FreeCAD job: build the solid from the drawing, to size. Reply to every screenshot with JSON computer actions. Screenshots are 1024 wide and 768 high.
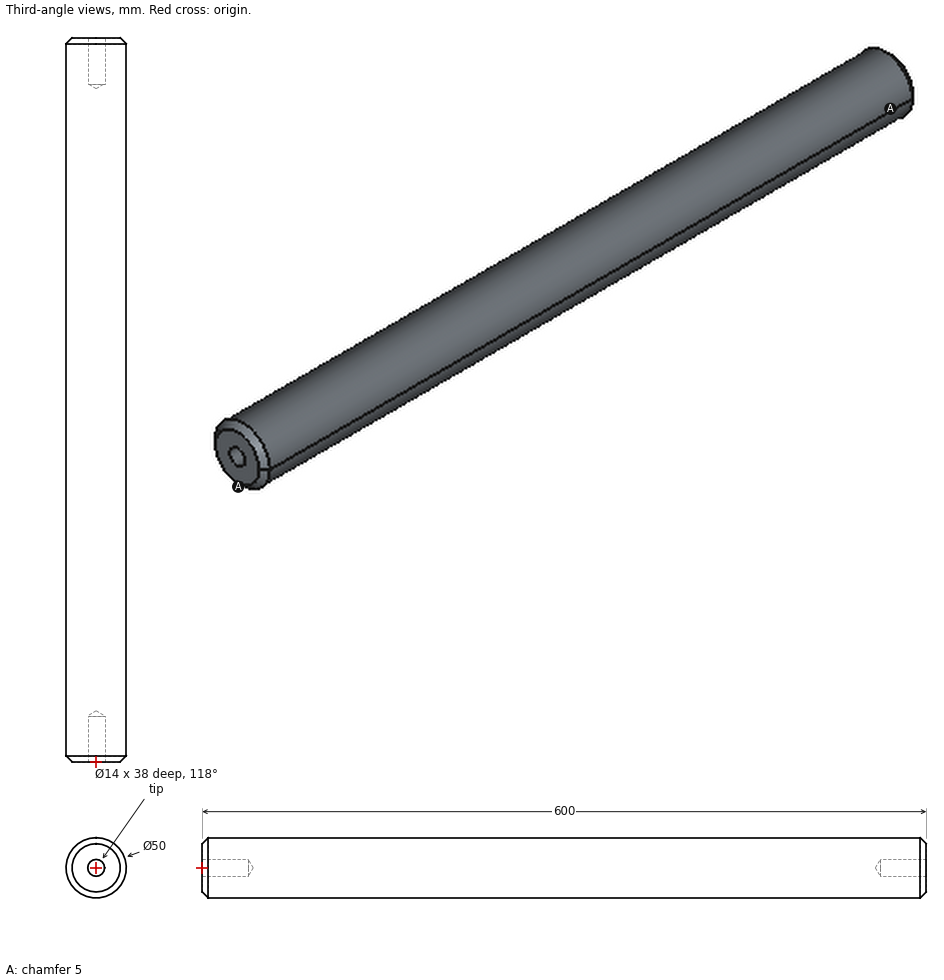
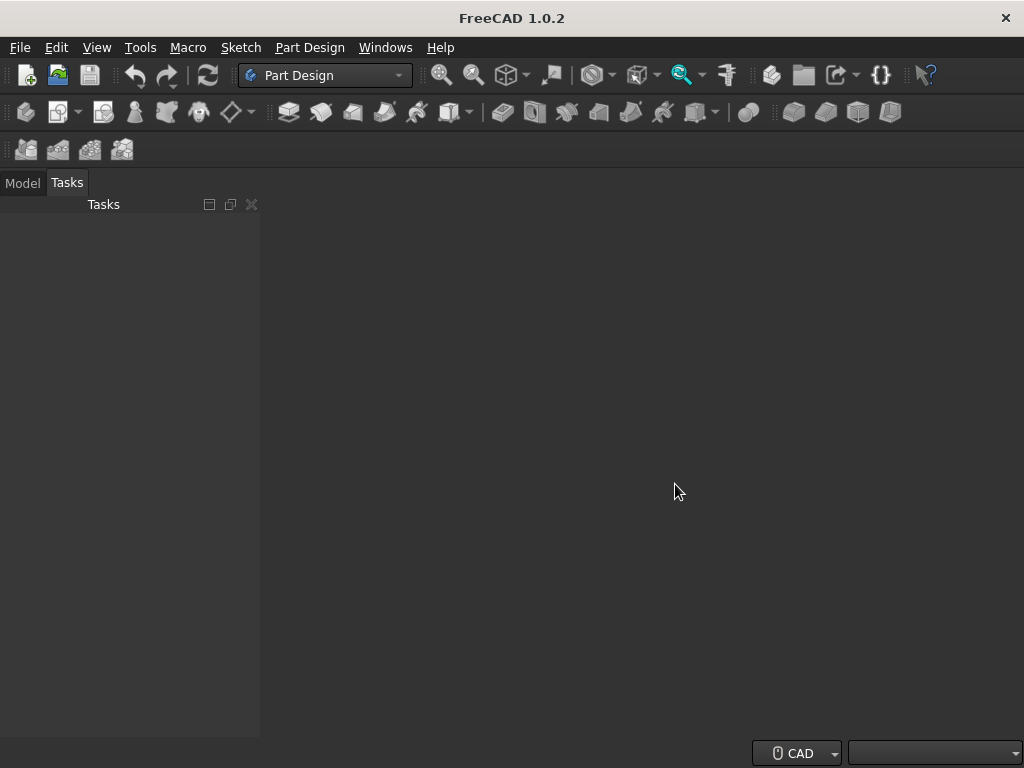
{"action": "left_click", "coordinate": [26, 76]}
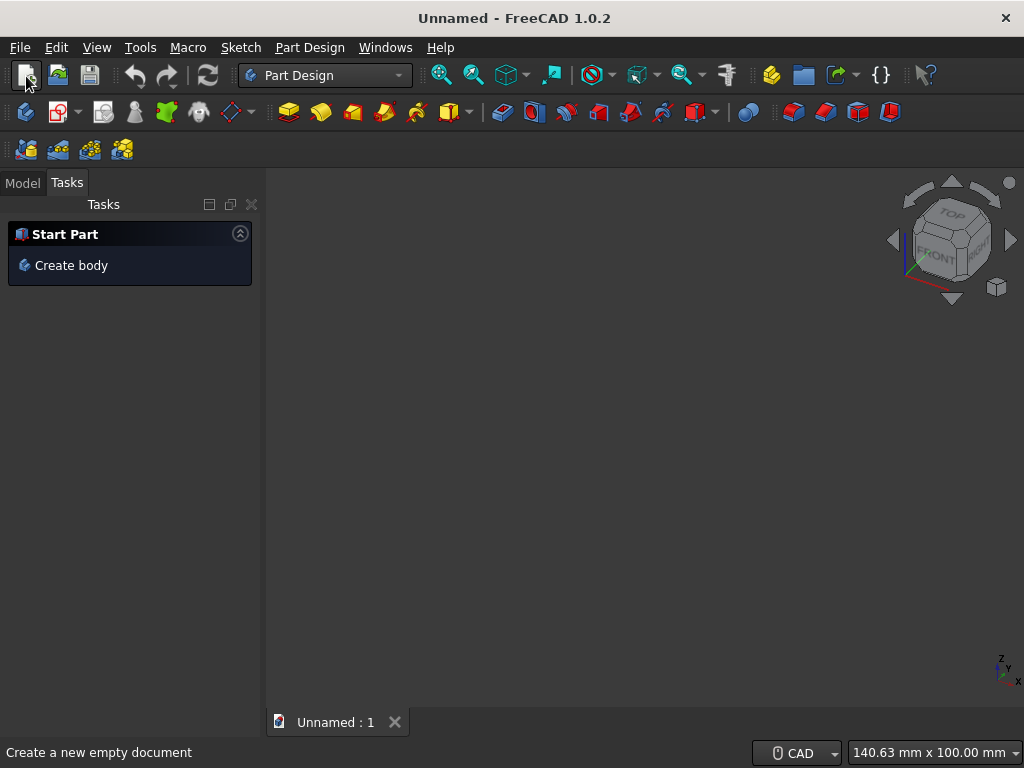
{"action": "left_click", "coordinate": [58, 112]}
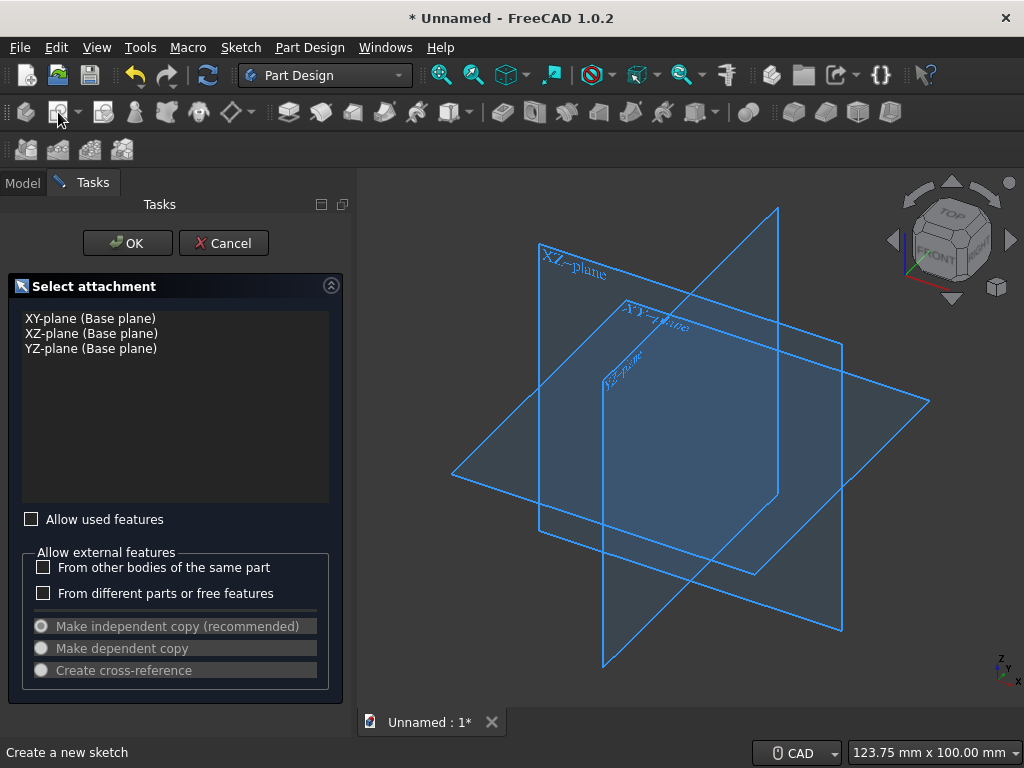
{"action": "left_click", "coordinate": [82, 334]}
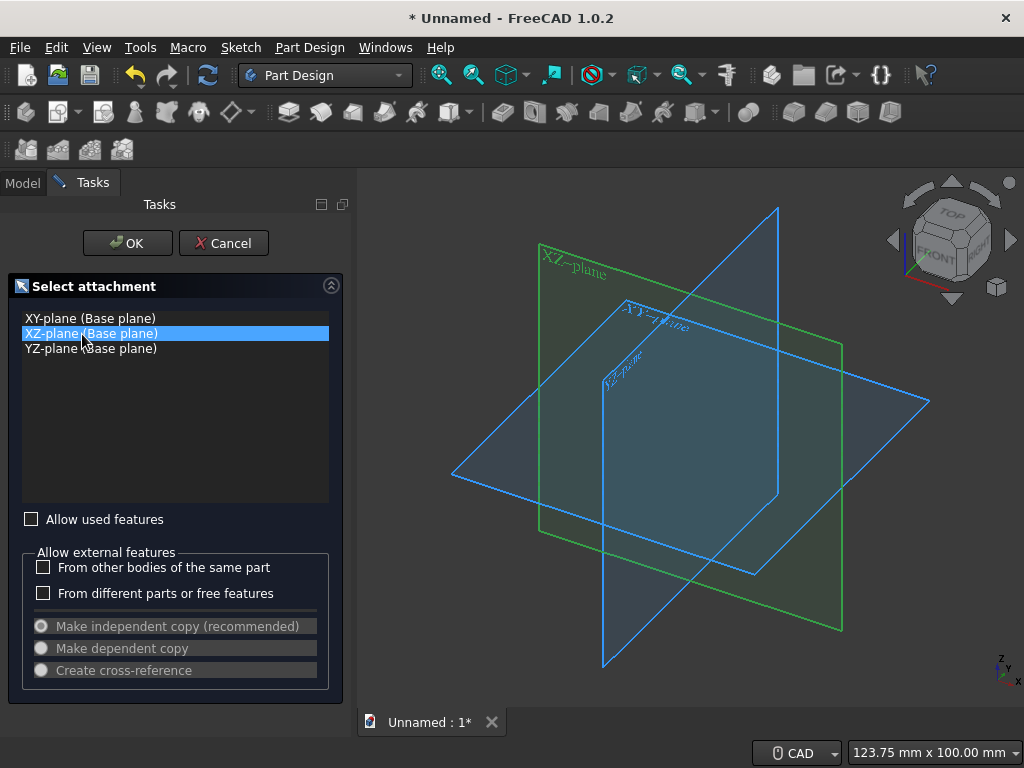
{"action": "left_click", "coordinate": [128, 243]}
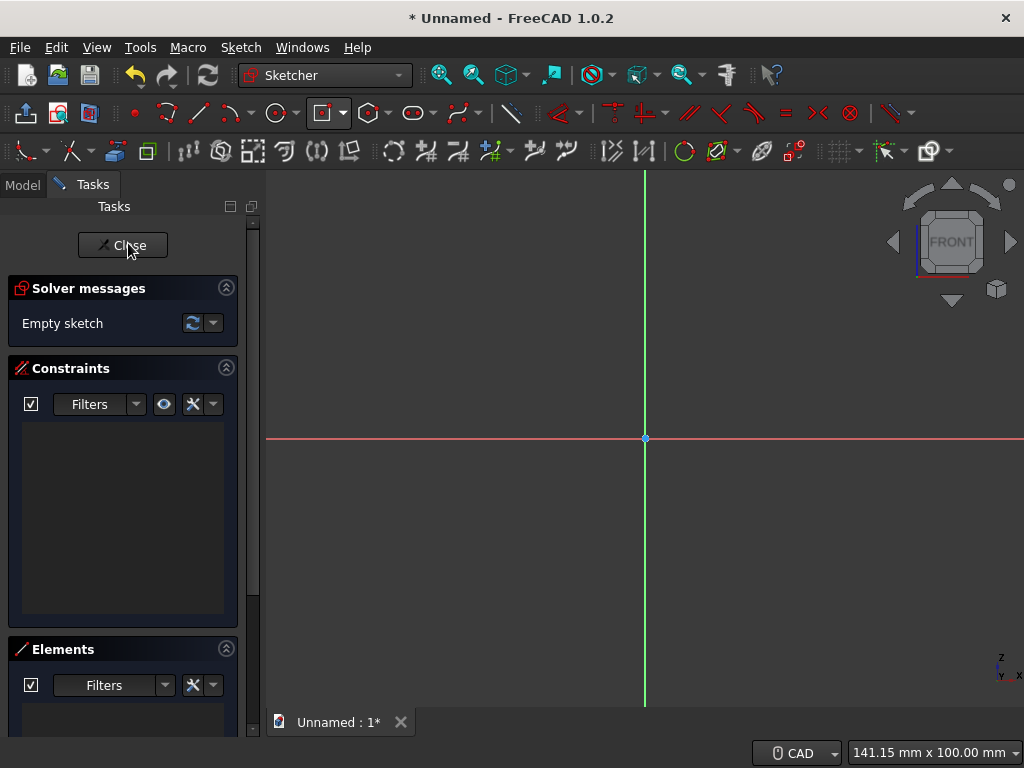
{"action": "left_click", "coordinate": [276, 114]}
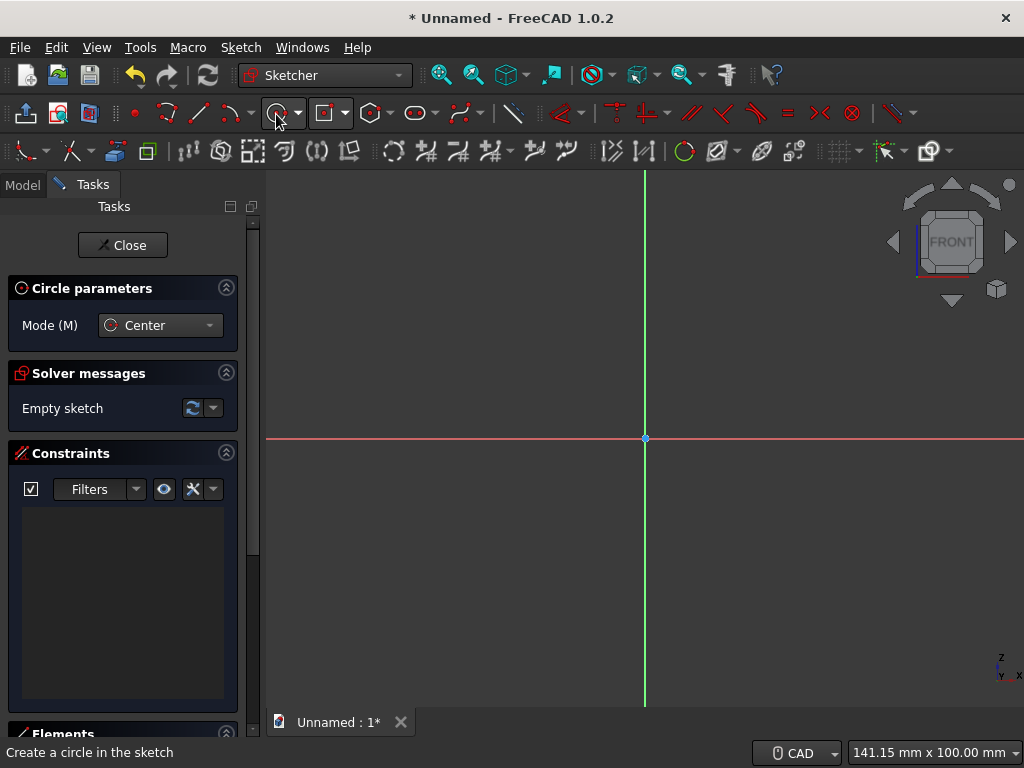
{"action": "left_click", "coordinate": [645, 438]}
{"action": "mouse_move", "coordinate": [740, 344]}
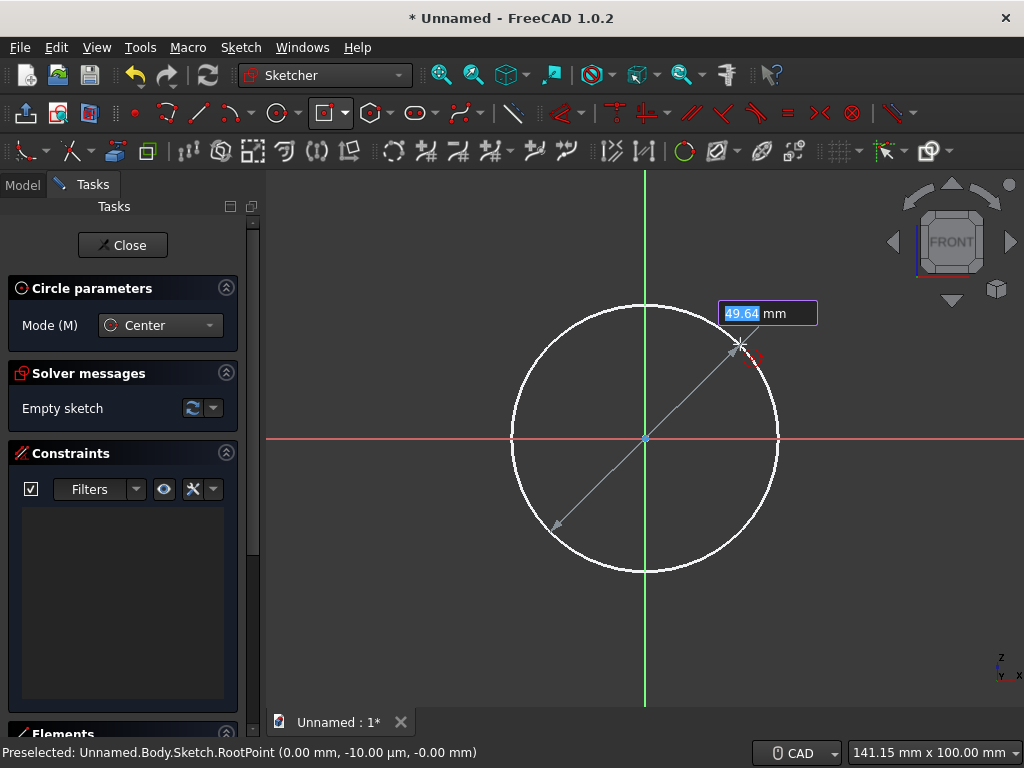
{"action": "type", "text": "50"}
{"action": "key", "text": "Return"}
{"action": "key", "text": "Escape"}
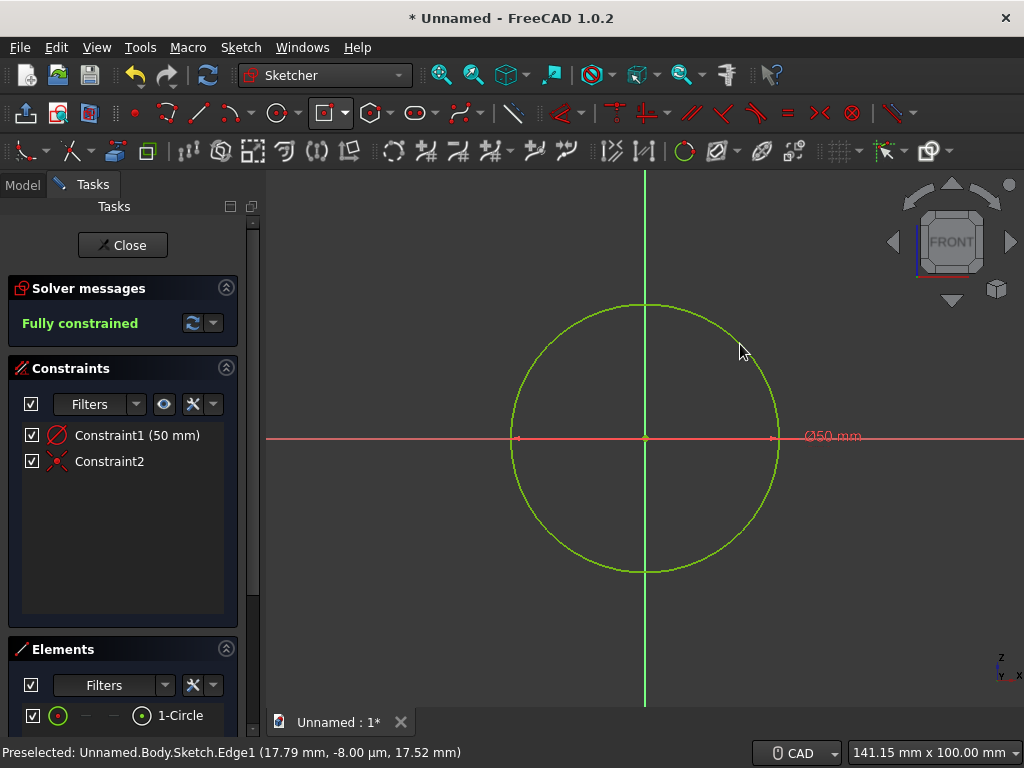
{"action": "left_click", "coordinate": [123, 245]}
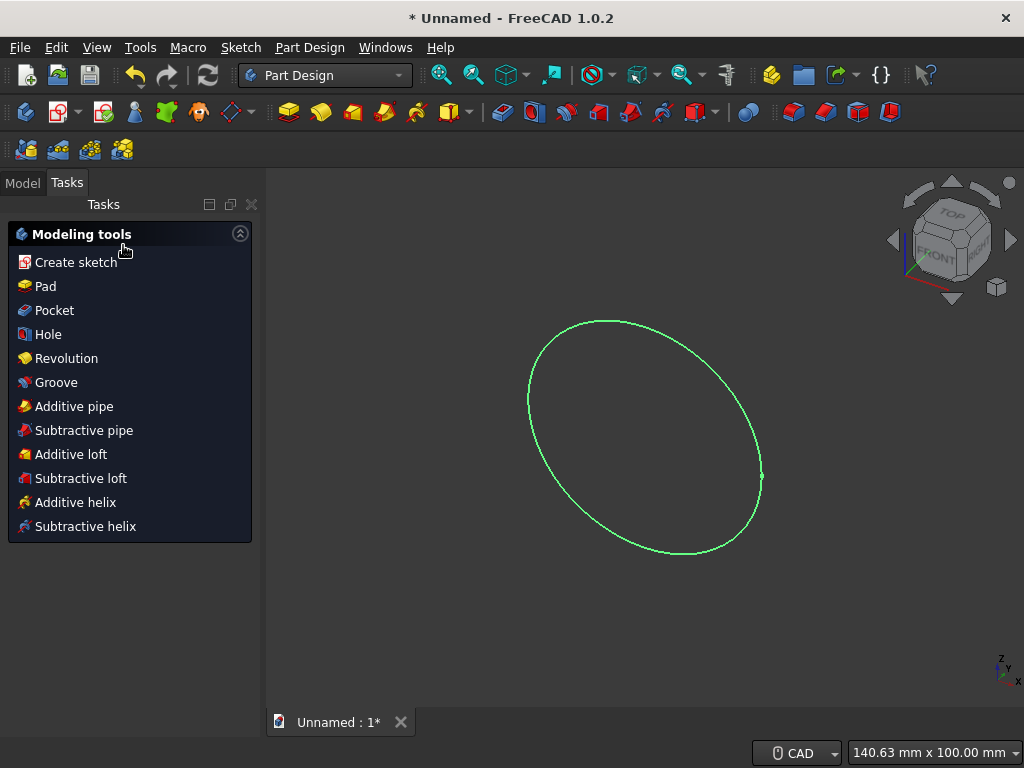
{"action": "left_click", "coordinate": [290, 112]}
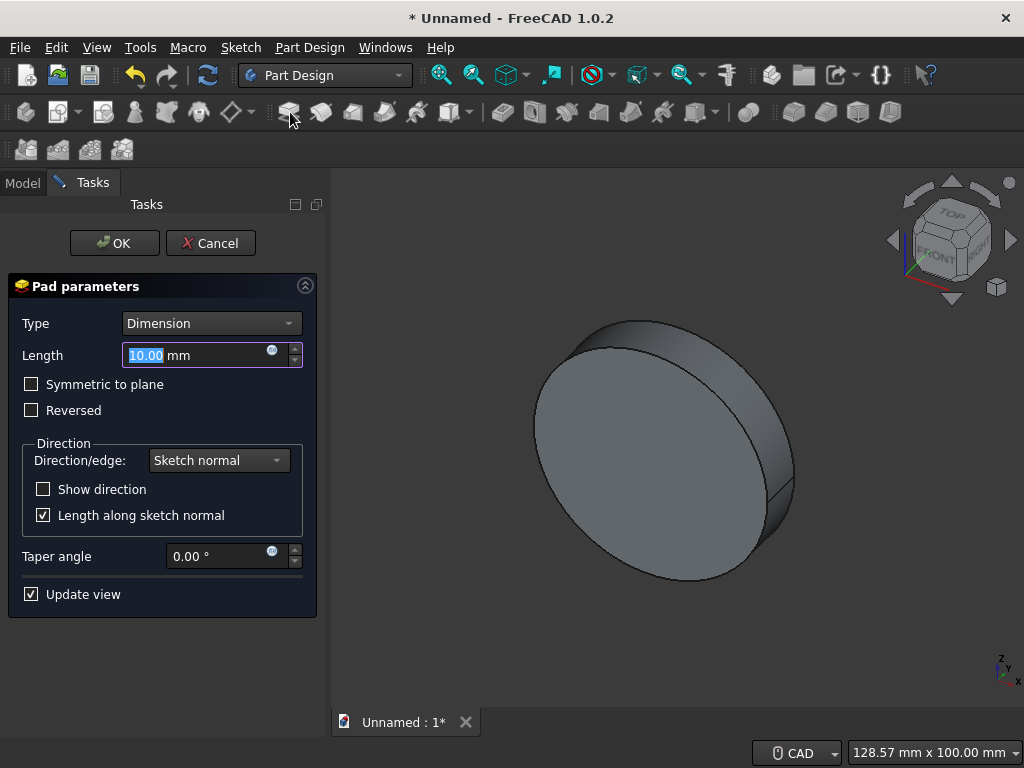
{"action": "type", "text": "600"}
{"action": "key", "text": "Tab"}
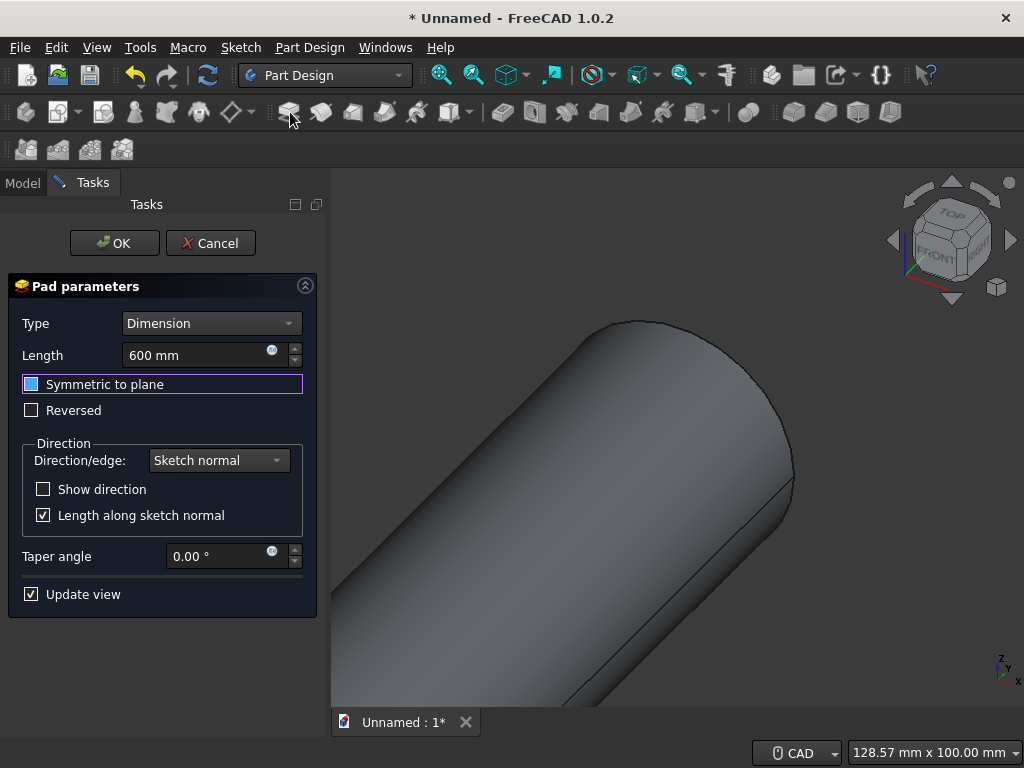
{"action": "left_click", "coordinate": [30, 410]}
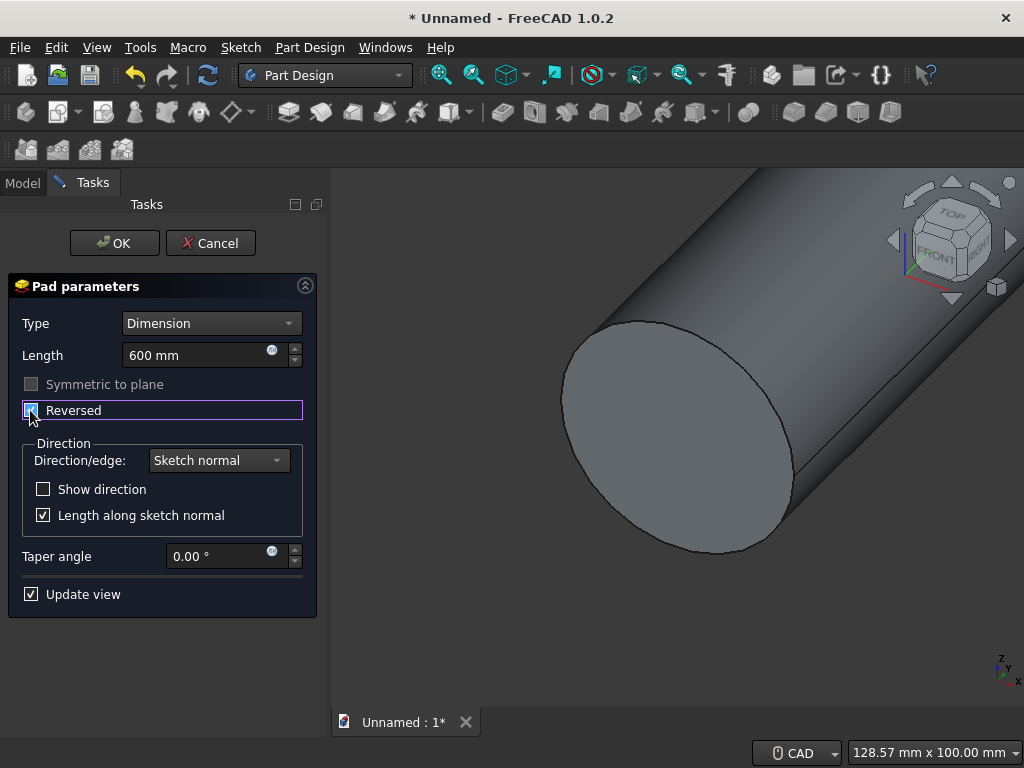
{"action": "left_click", "coordinate": [115, 243]}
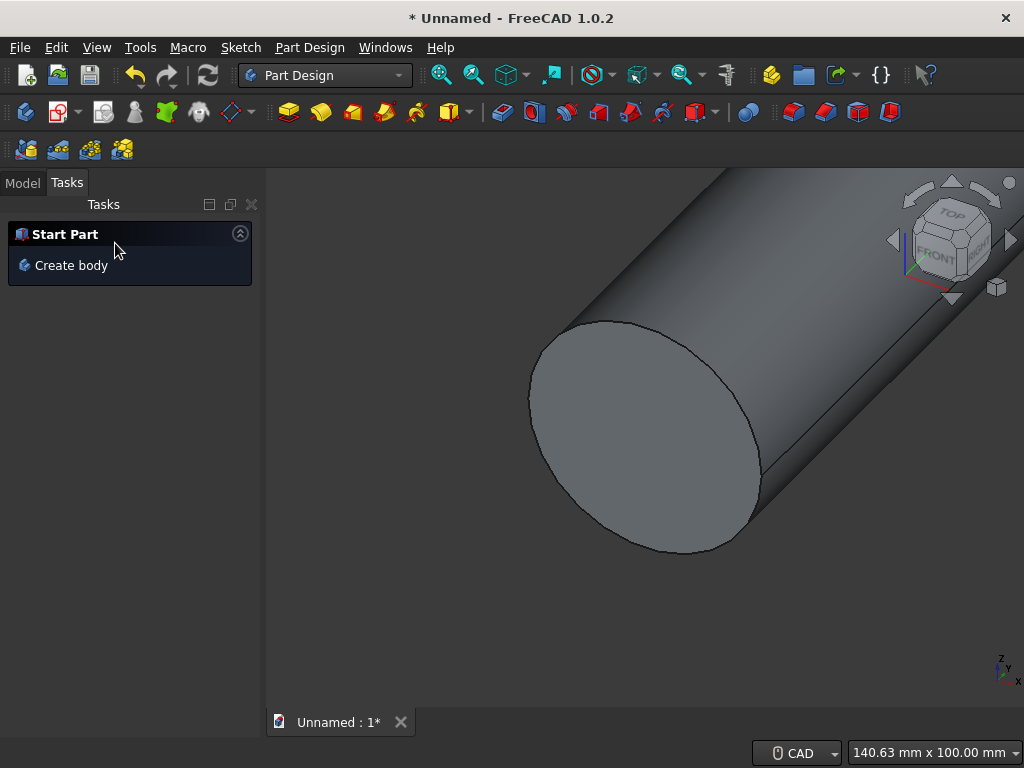
{"action": "key", "text": "v f"}